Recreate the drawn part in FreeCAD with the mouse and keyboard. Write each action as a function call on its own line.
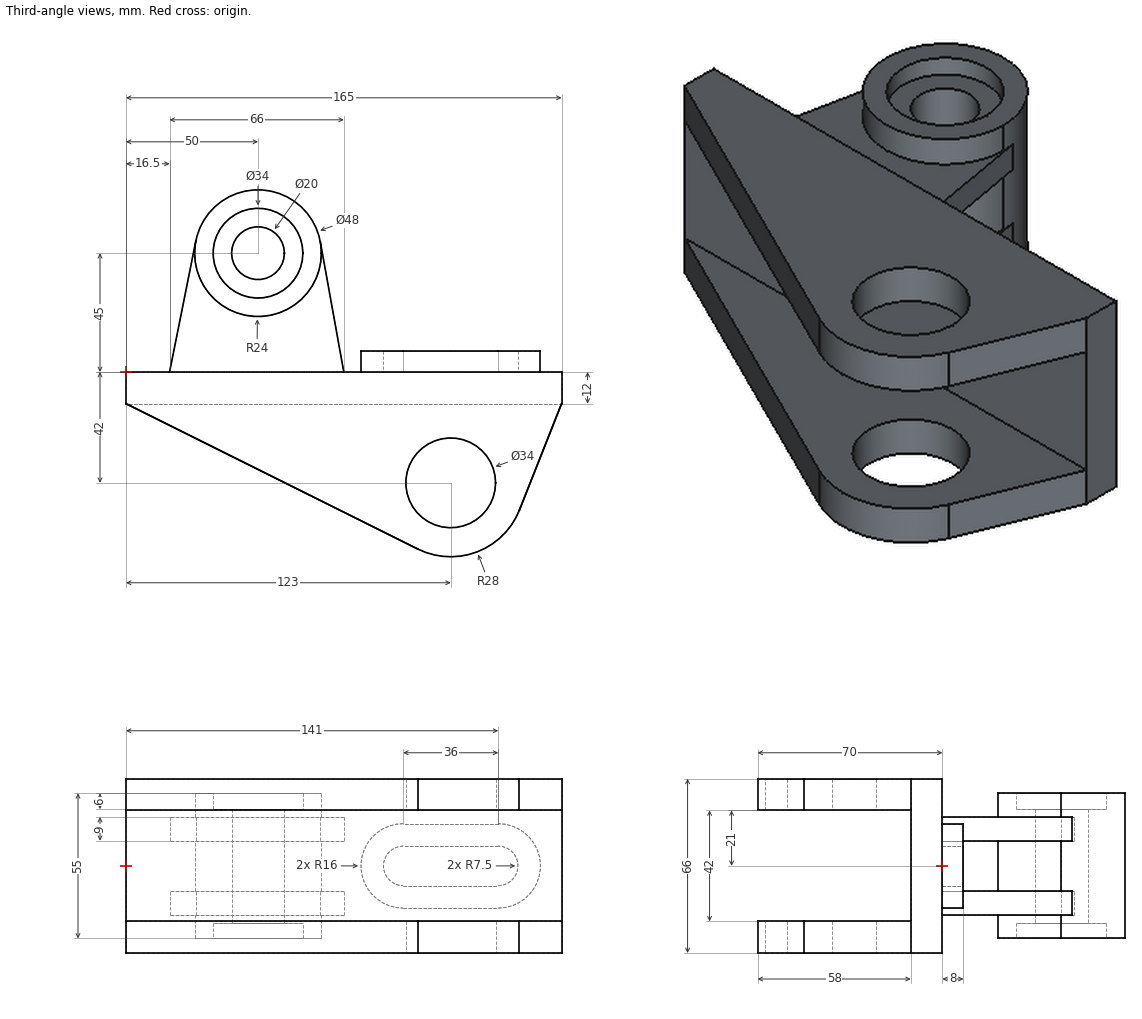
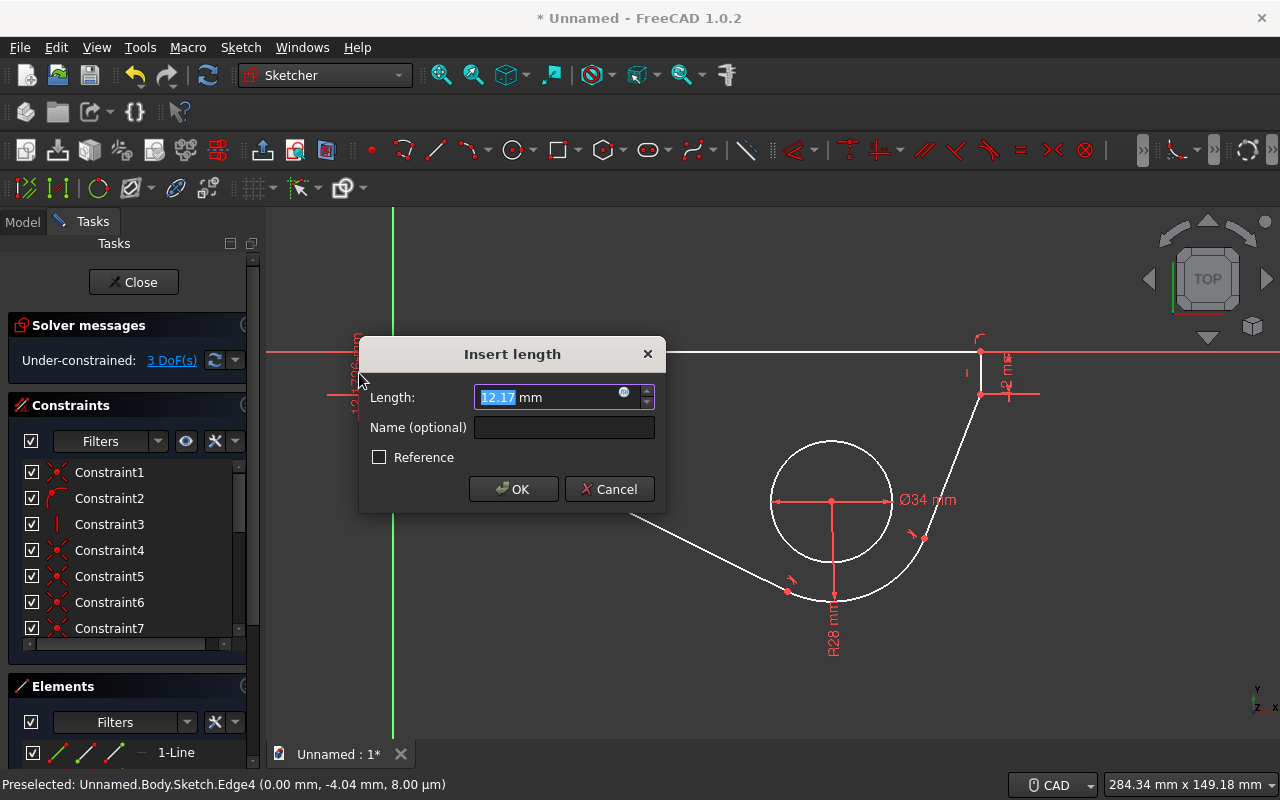
text(12)
key(Return)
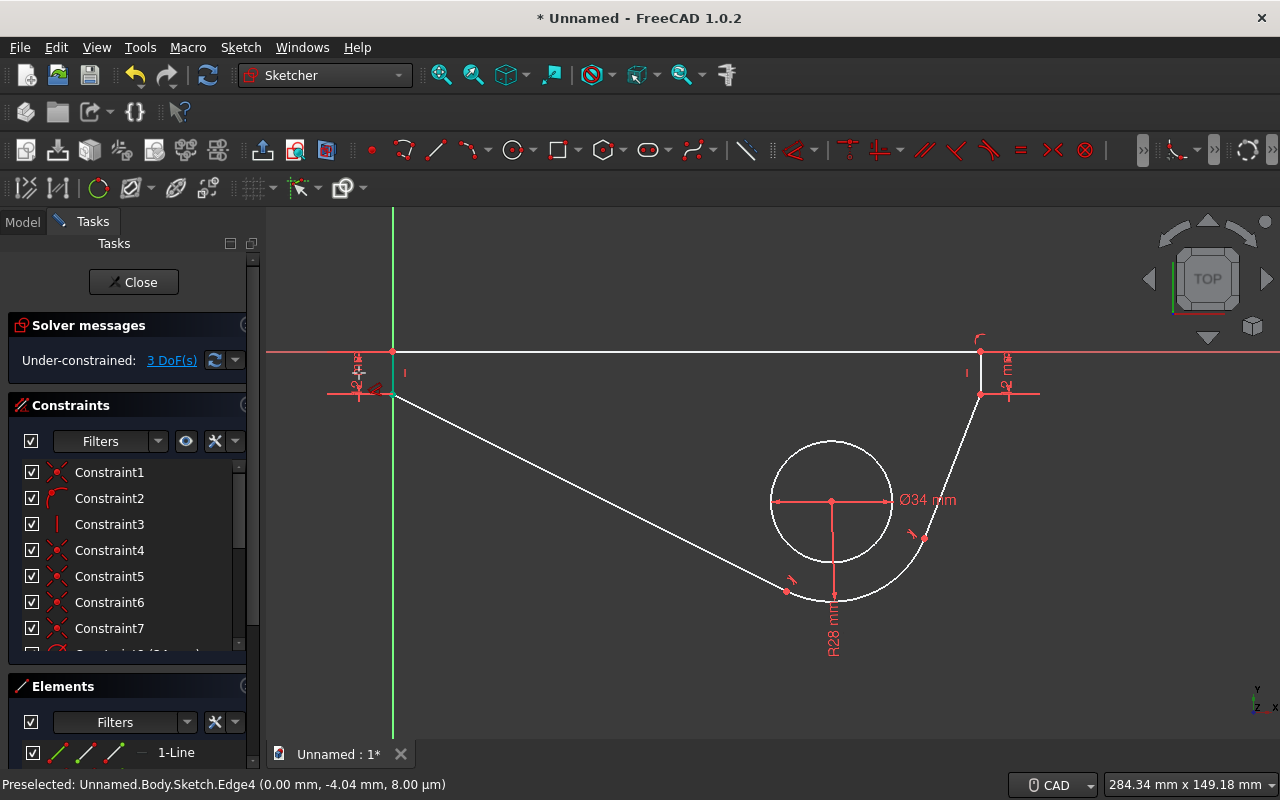
click(832, 502)
click(359, 427)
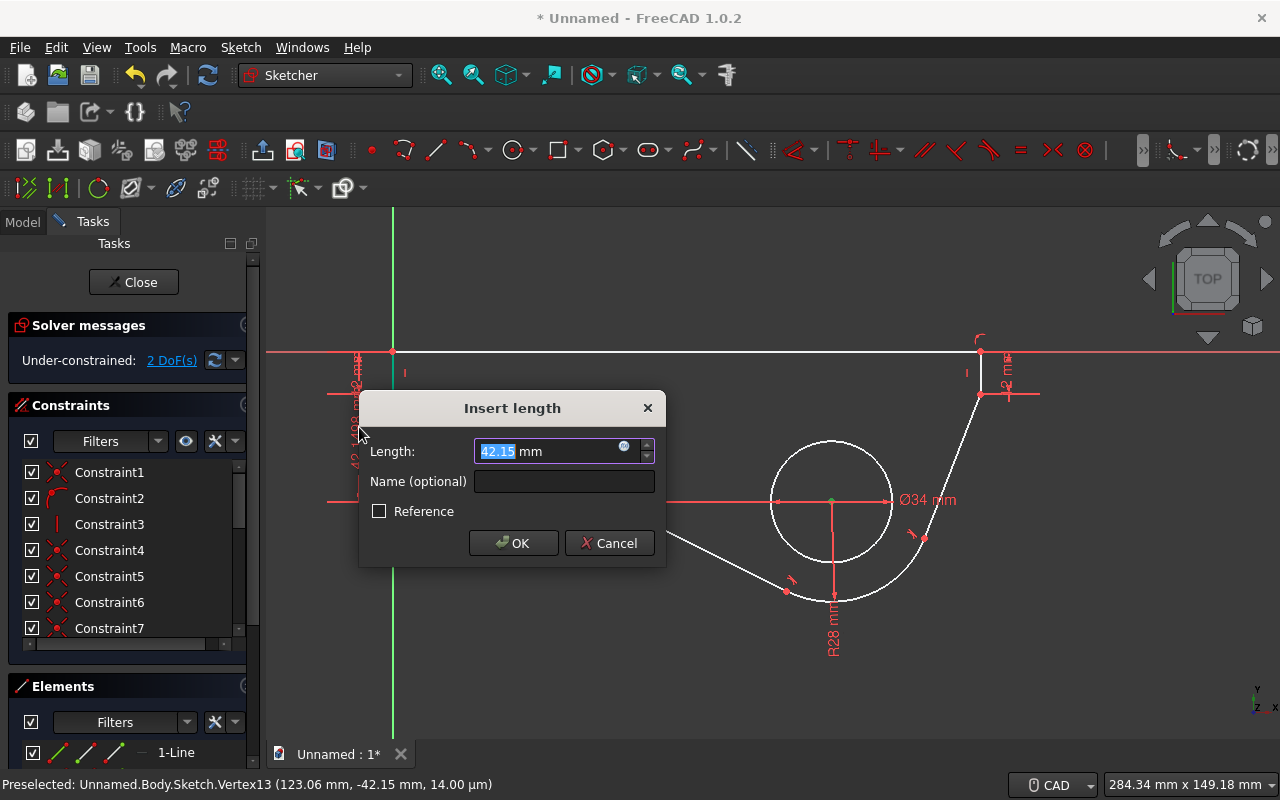
text(42)
key(Return)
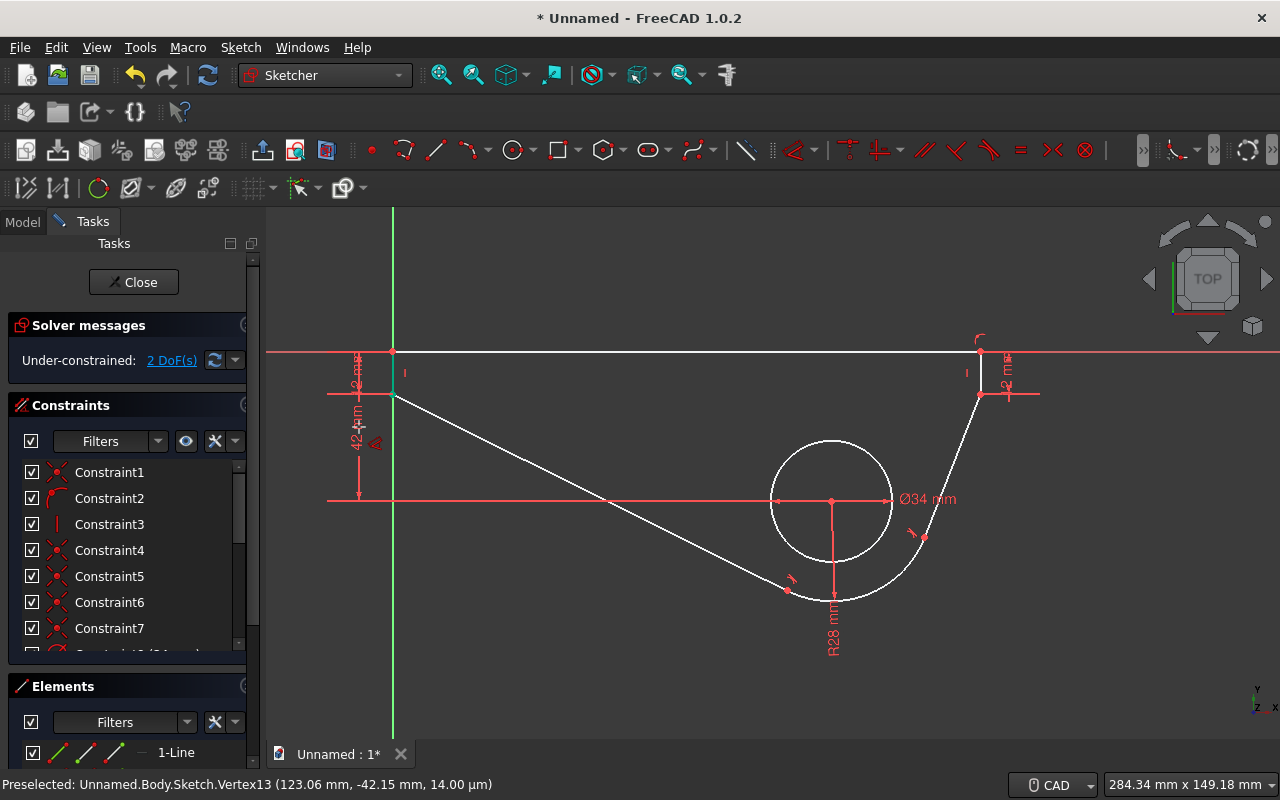
click(804, 352)
click(687, 318)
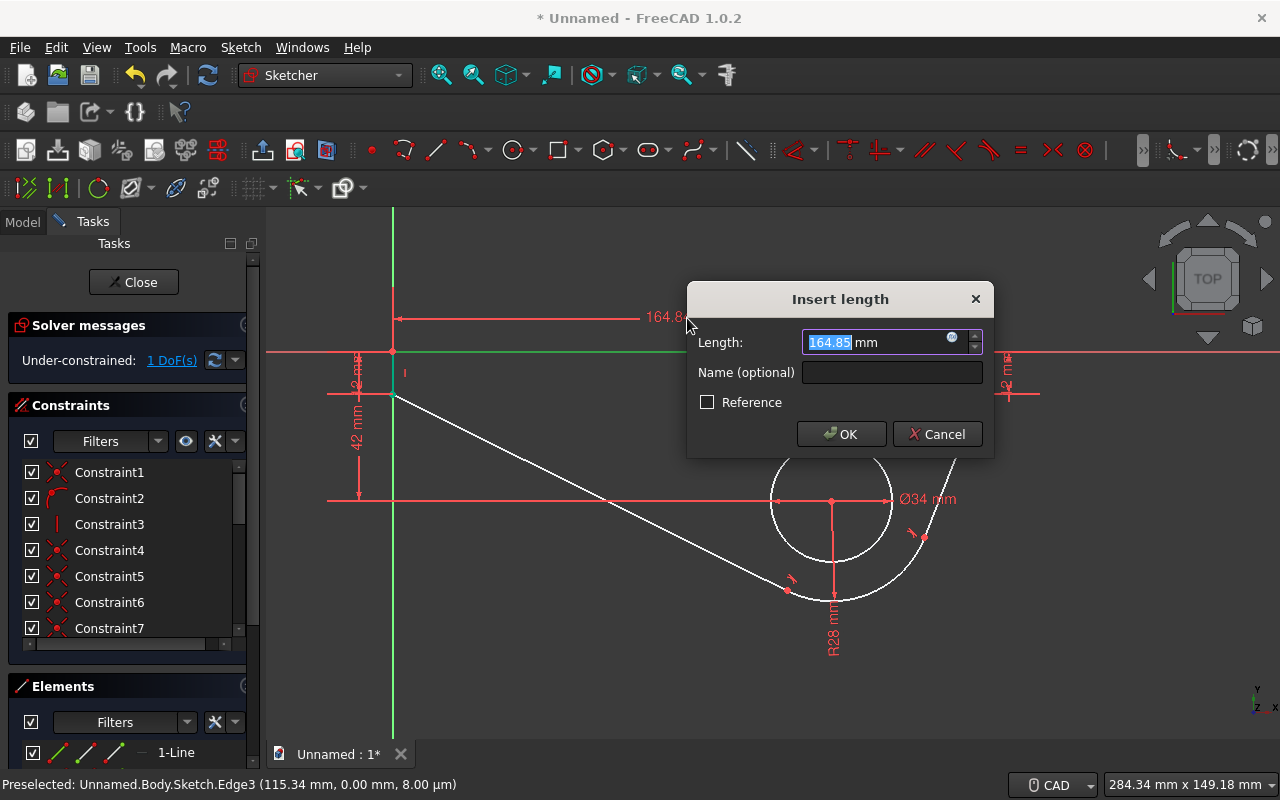
text(165)
key(Return)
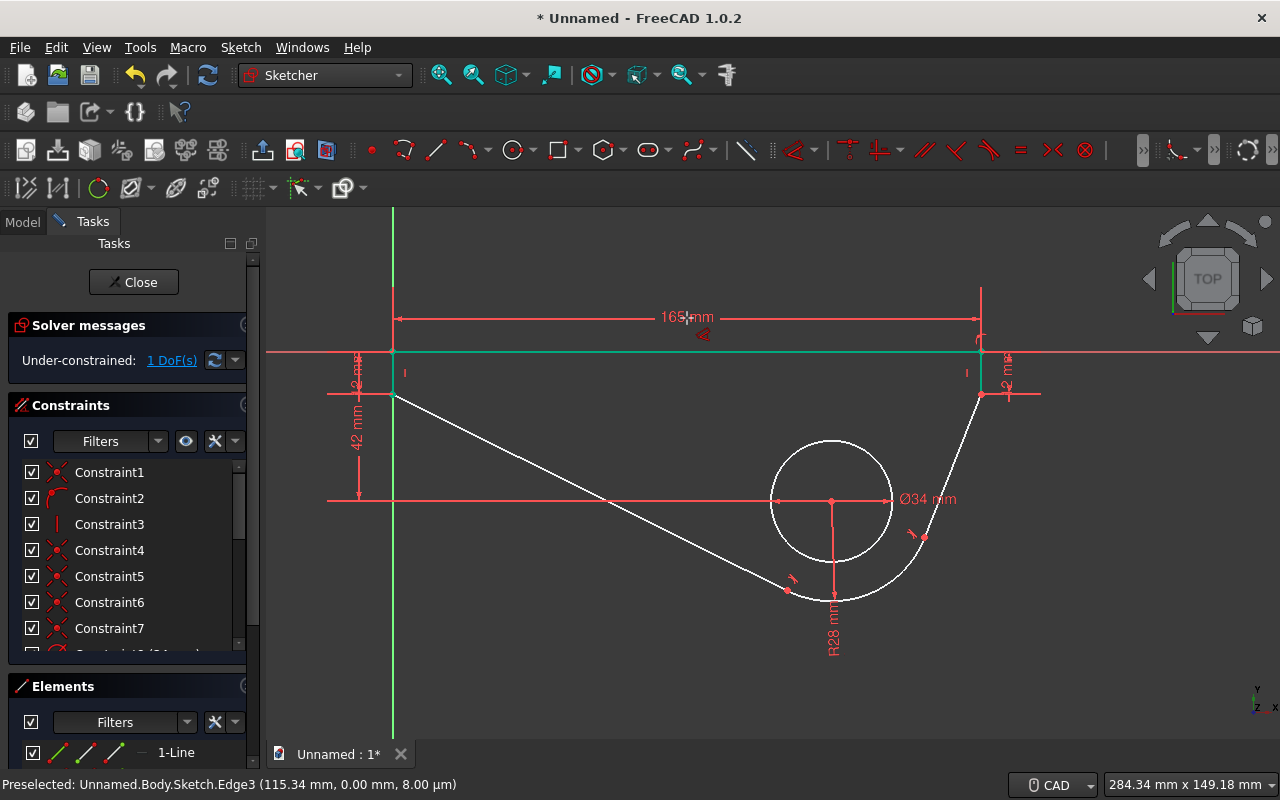
click(832, 501)
click(612, 318)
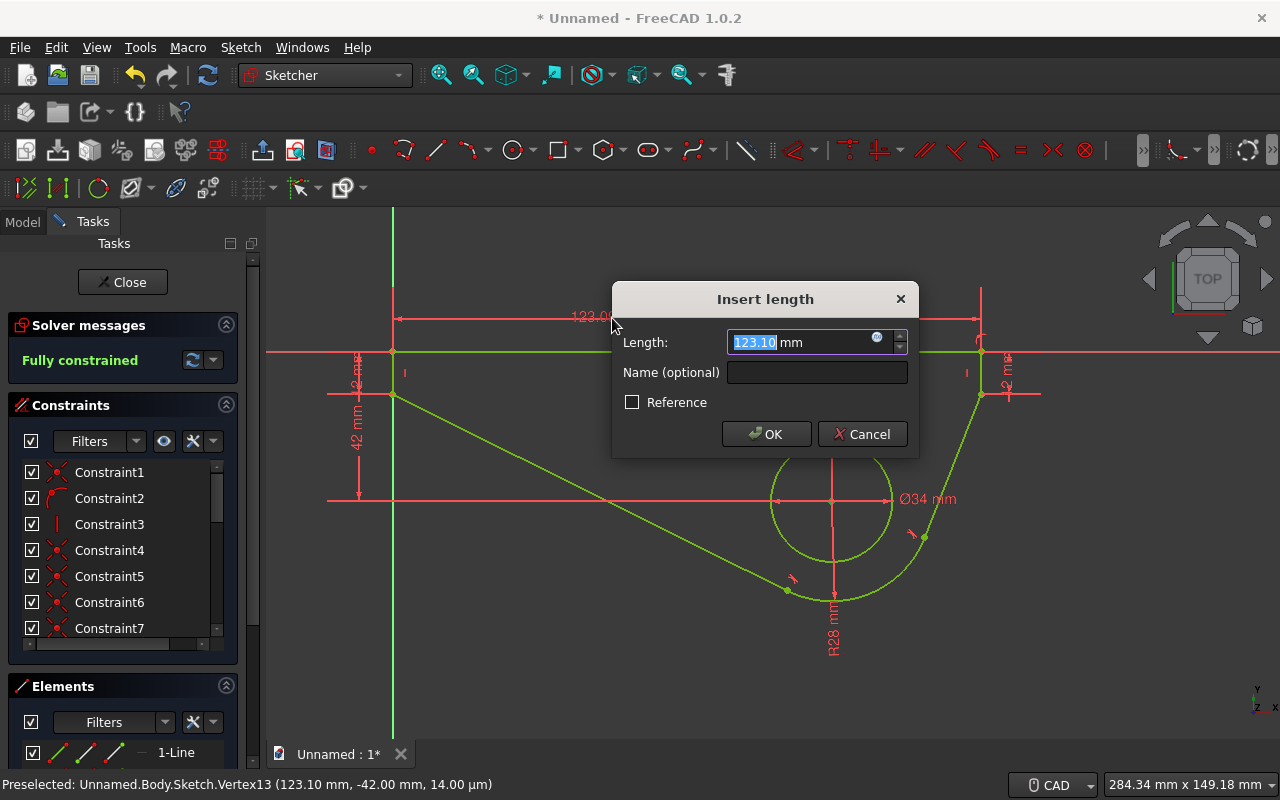
text(123)
key(Return)
key(Escape)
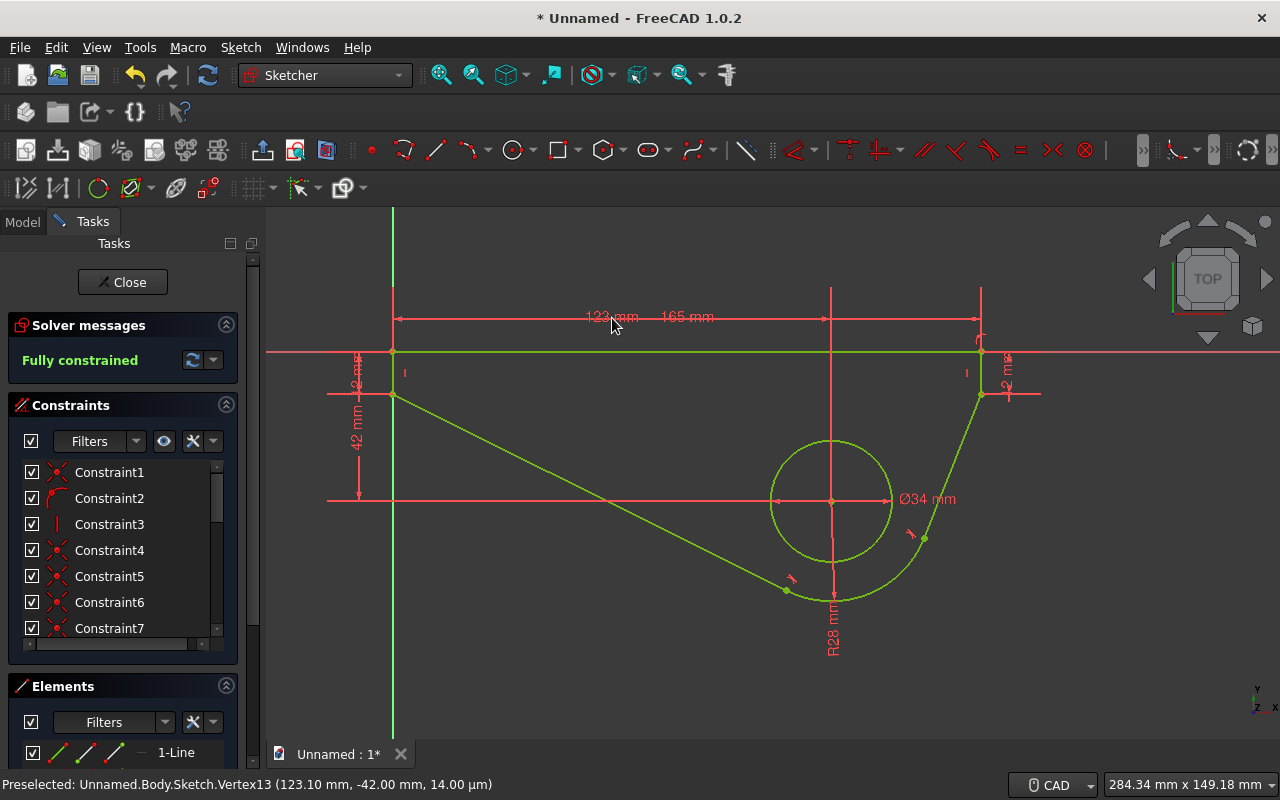
click(123, 282)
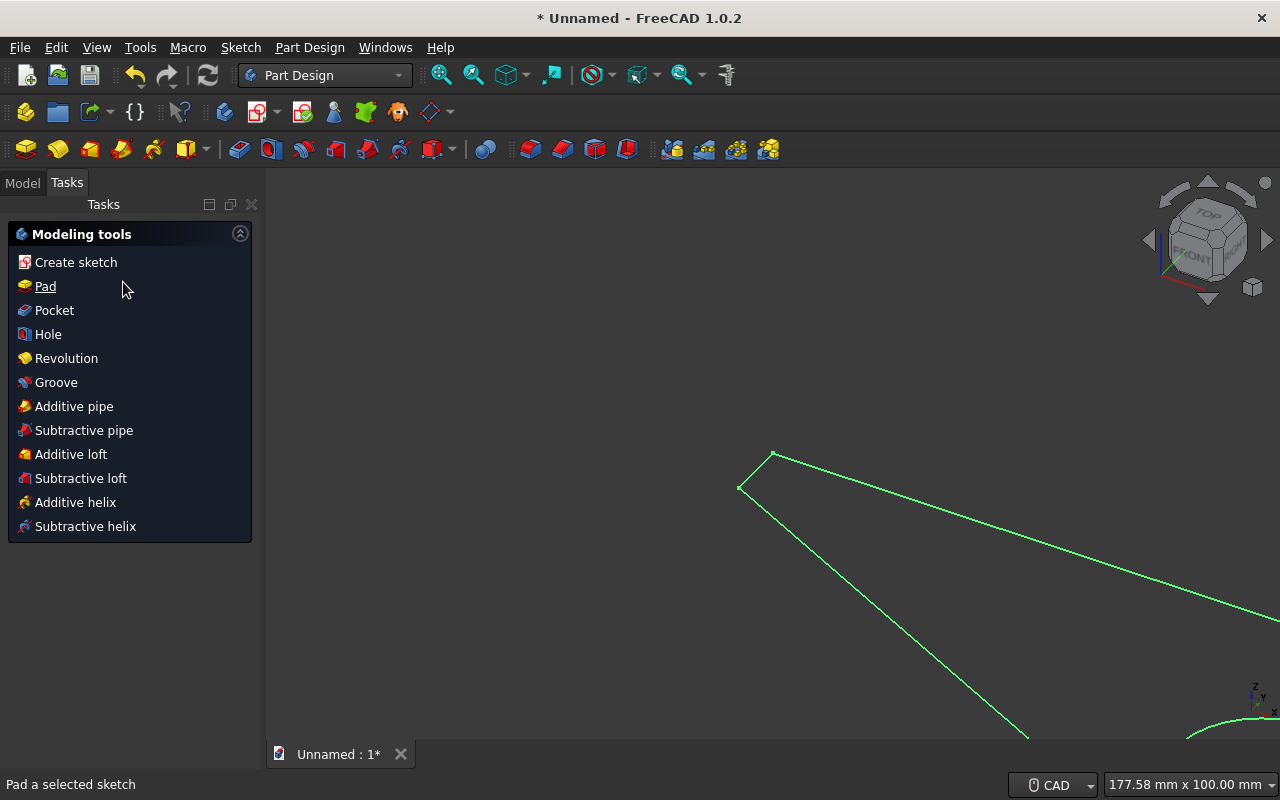
click(26, 150)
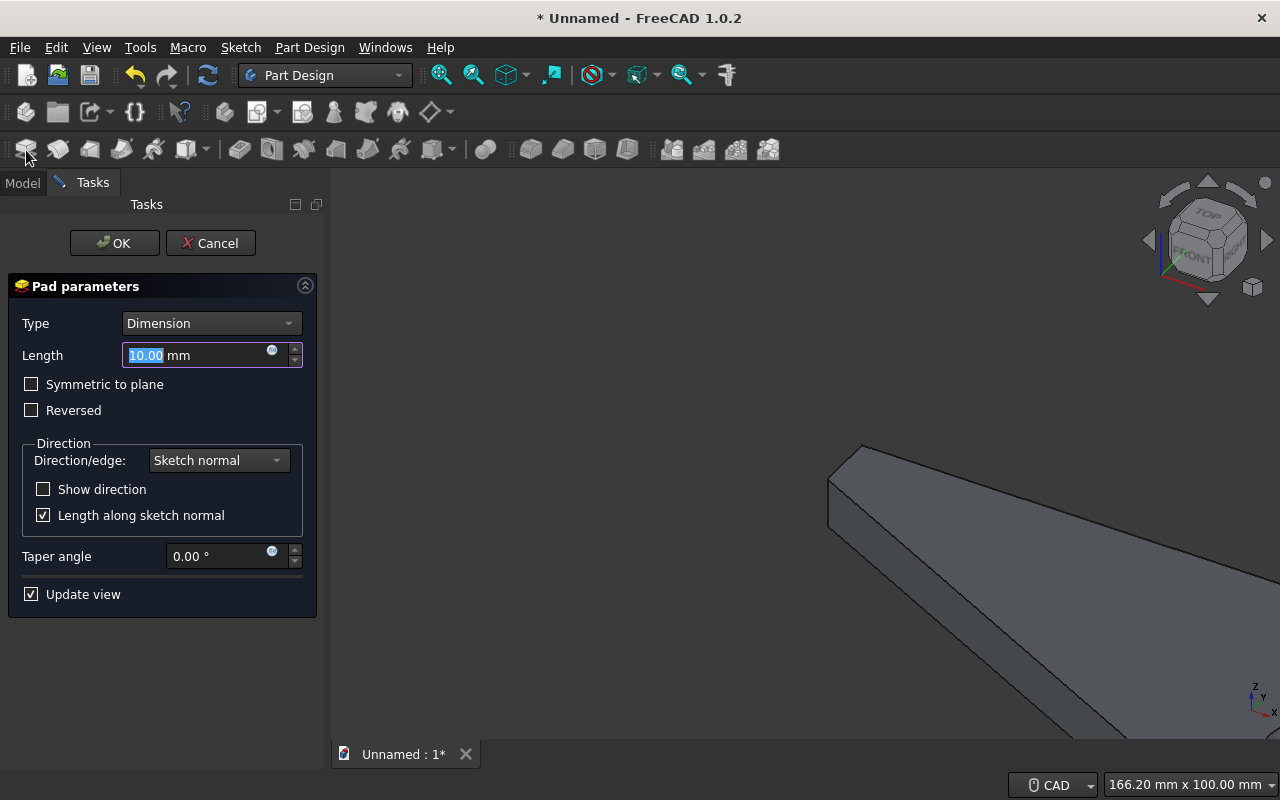
text(66)
key(Tab)